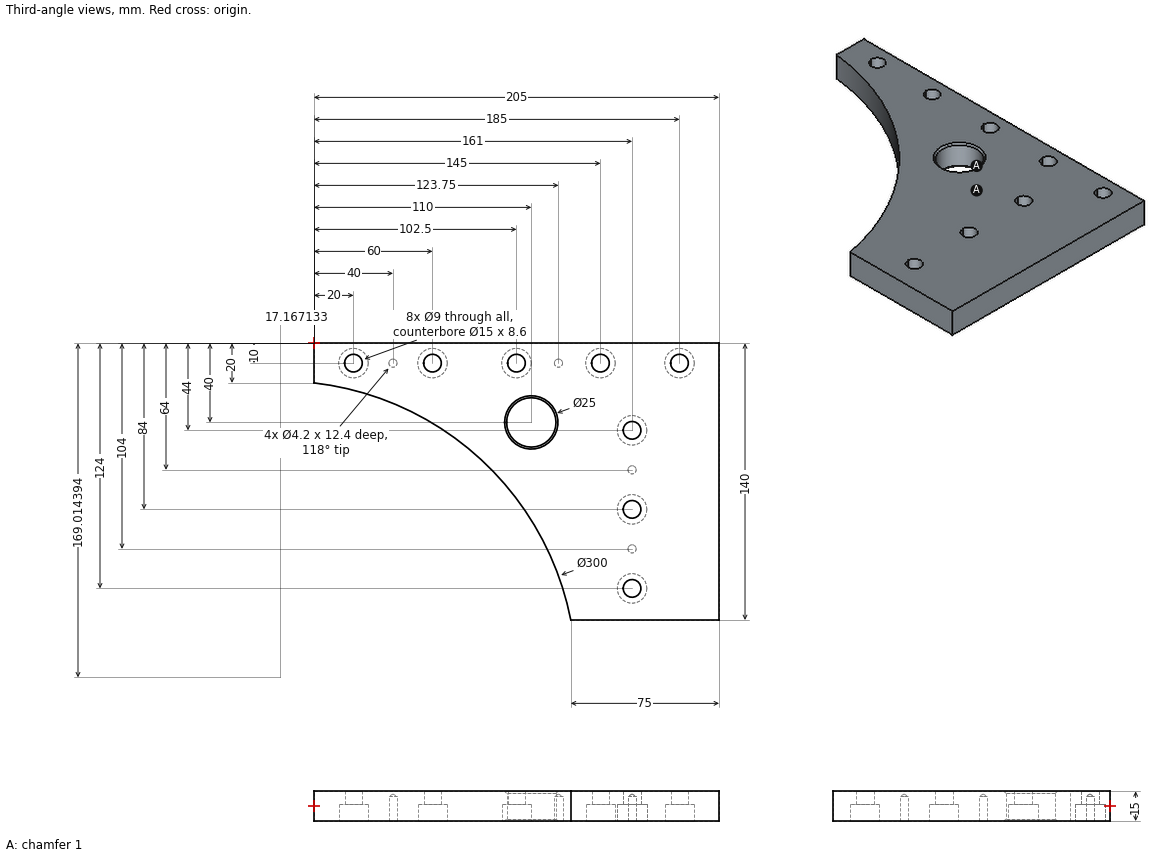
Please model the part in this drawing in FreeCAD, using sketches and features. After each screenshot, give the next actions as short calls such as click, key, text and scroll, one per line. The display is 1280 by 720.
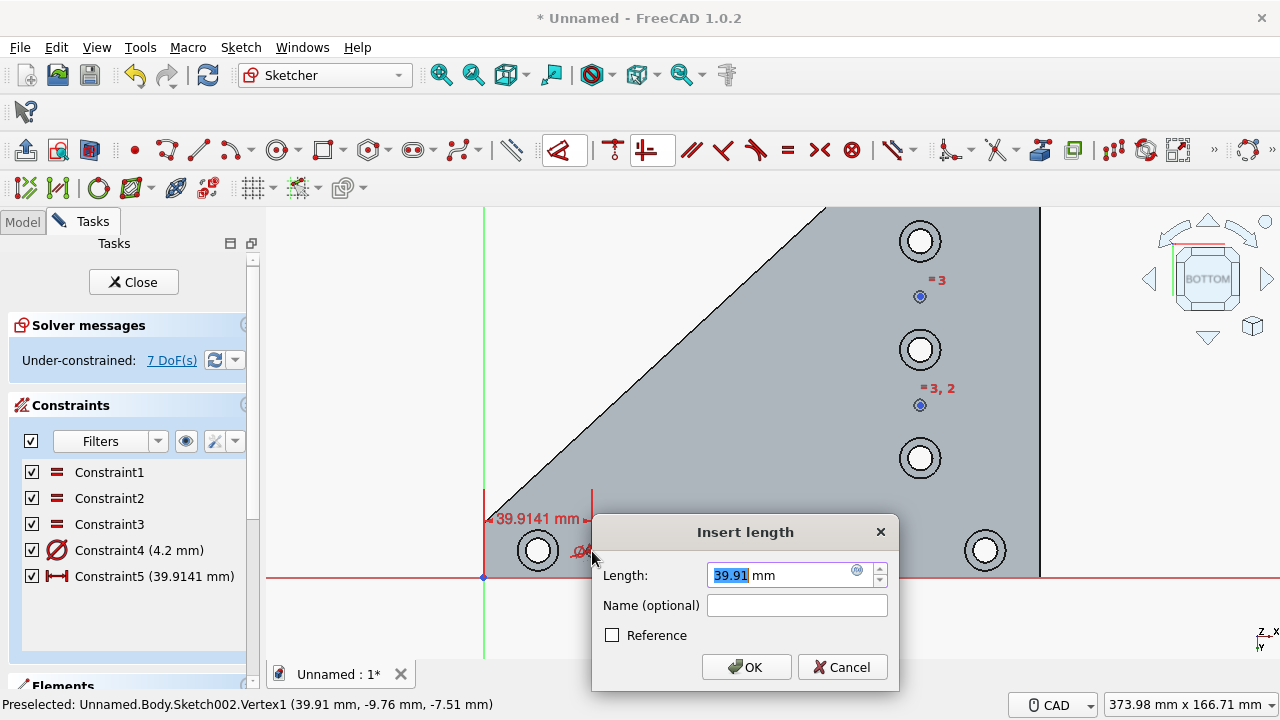
text(40)
key(Return)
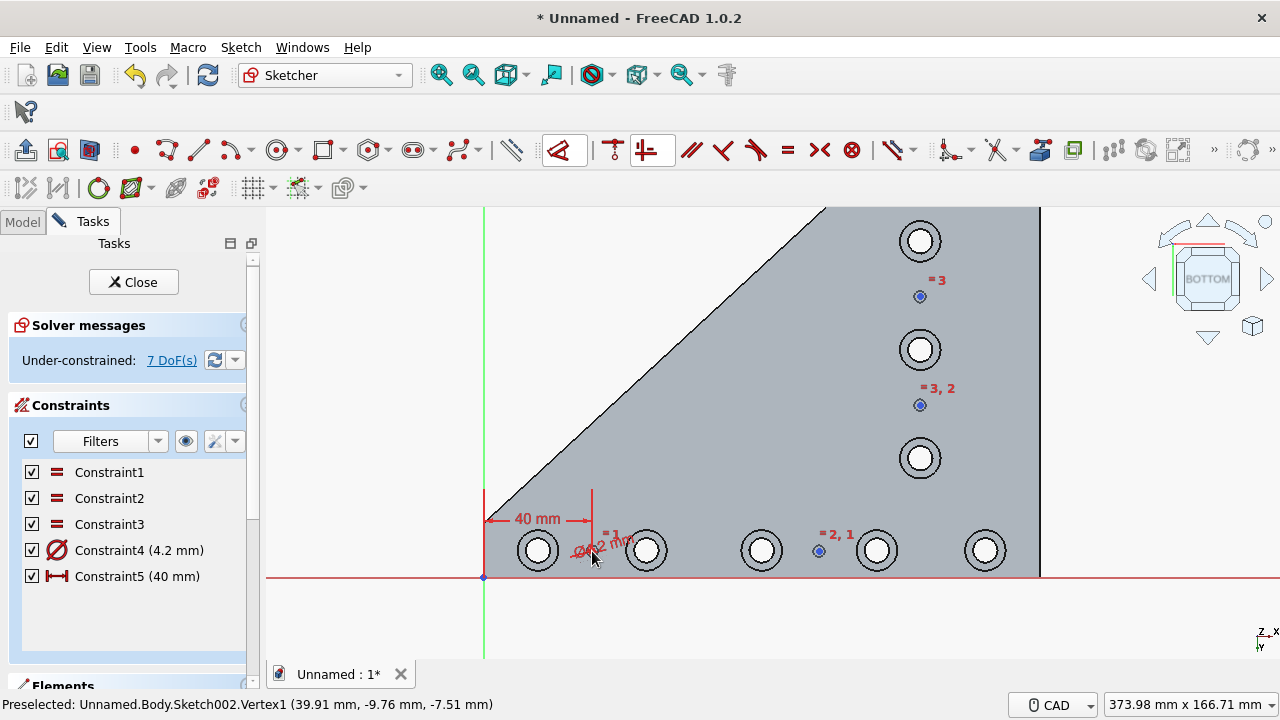
scroll(592, 551, up, 2)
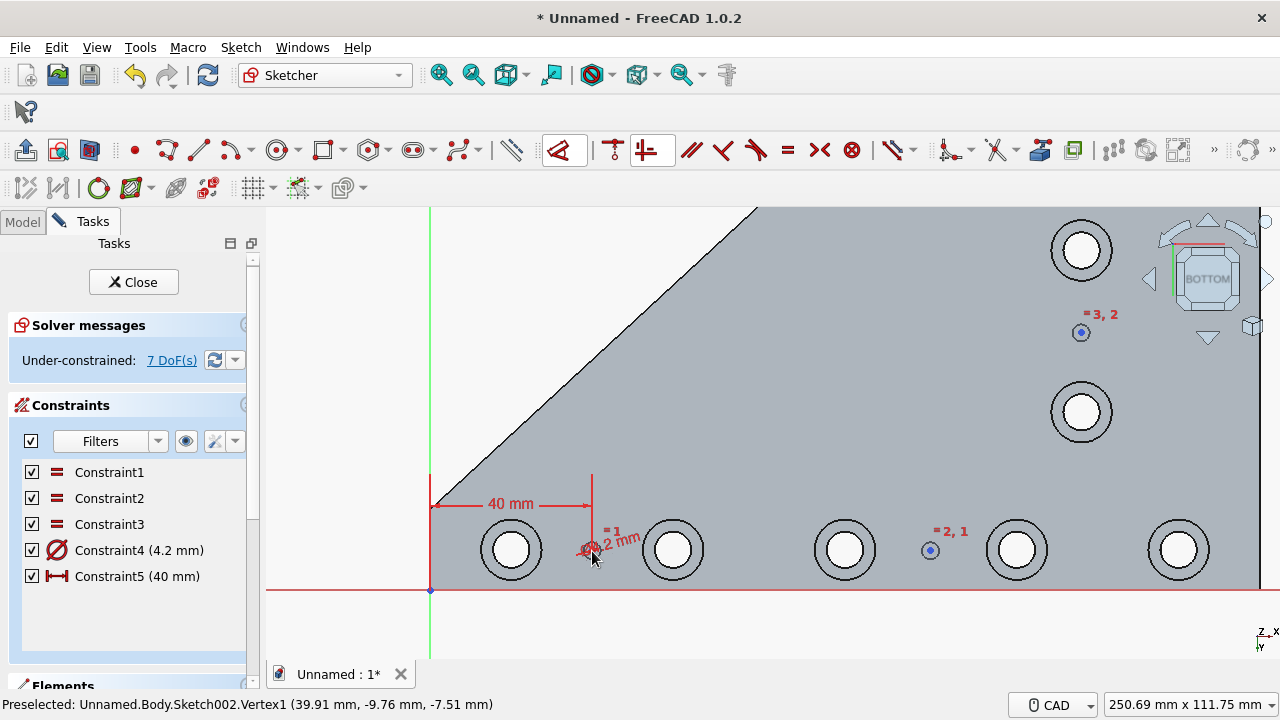
click(592, 551)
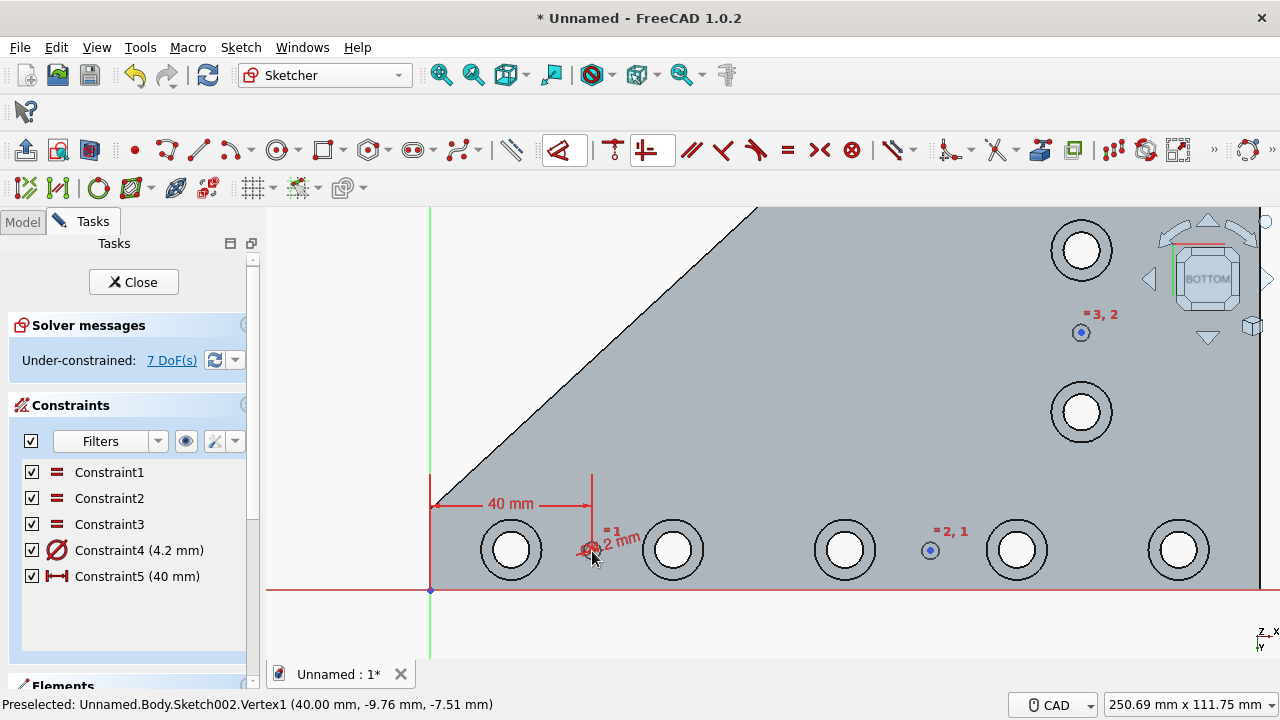
click(582, 150)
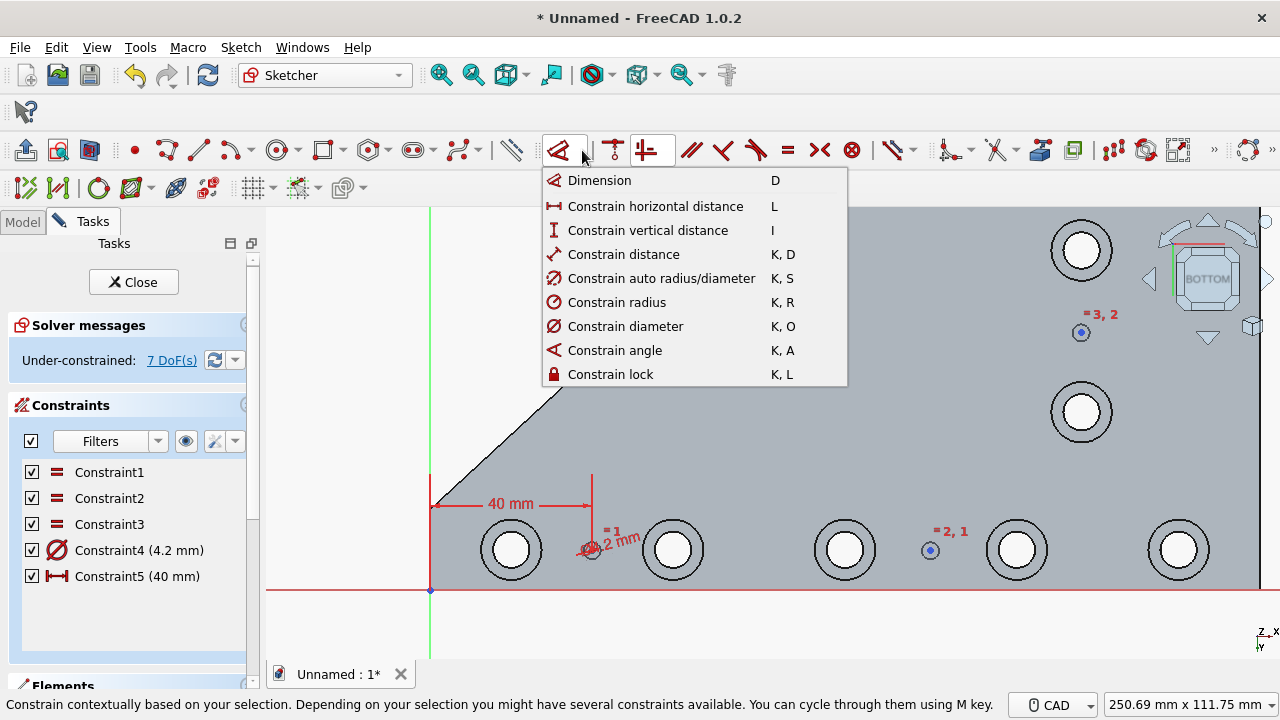
click(695, 230)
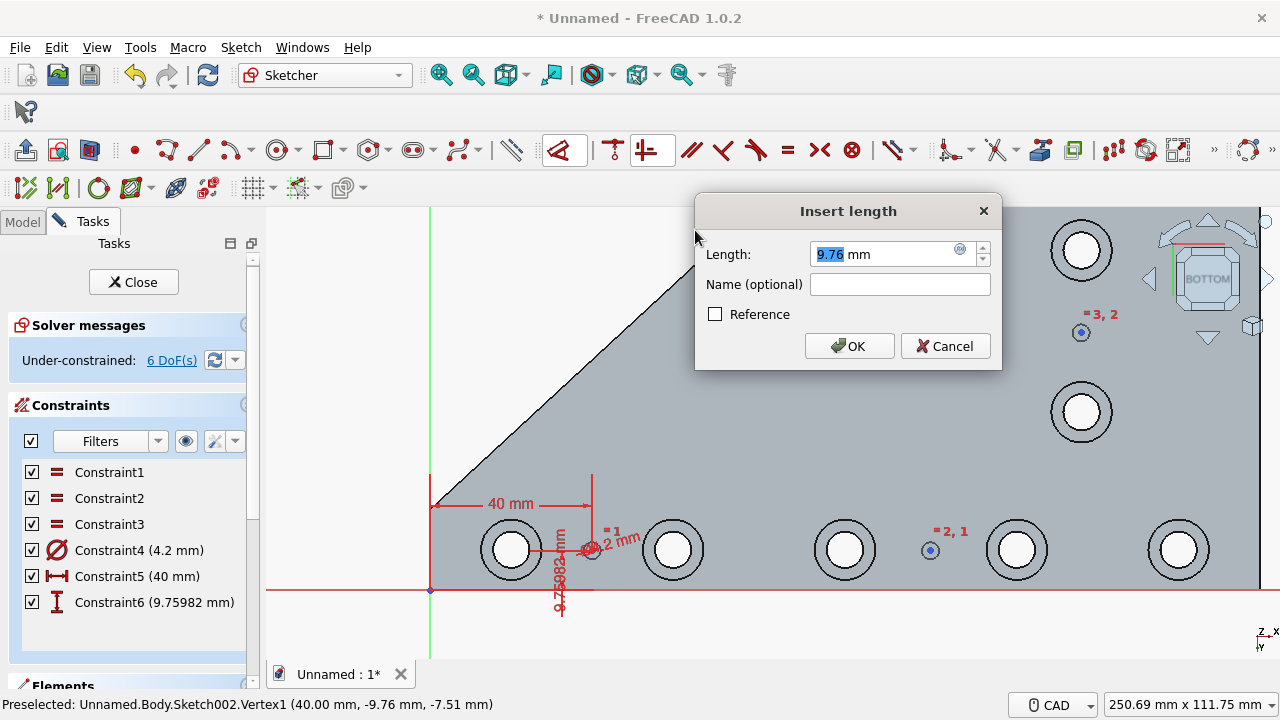
text(10)
key(Return)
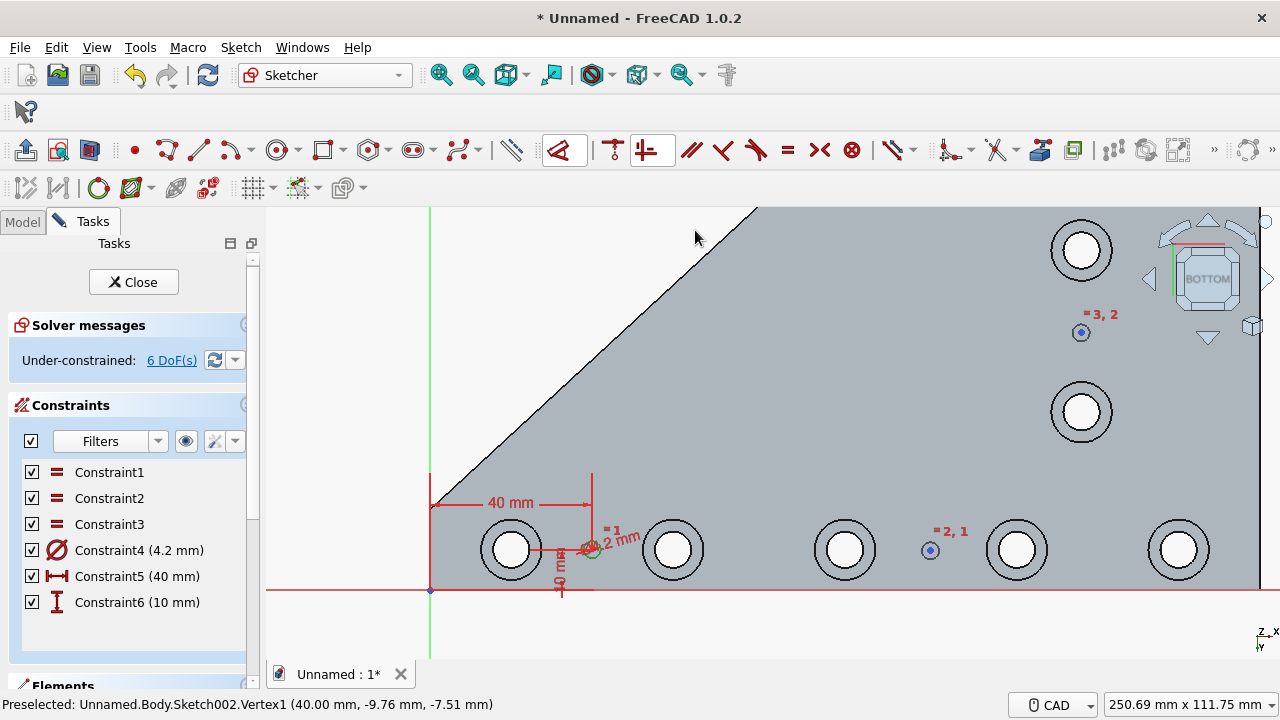
click(930, 551)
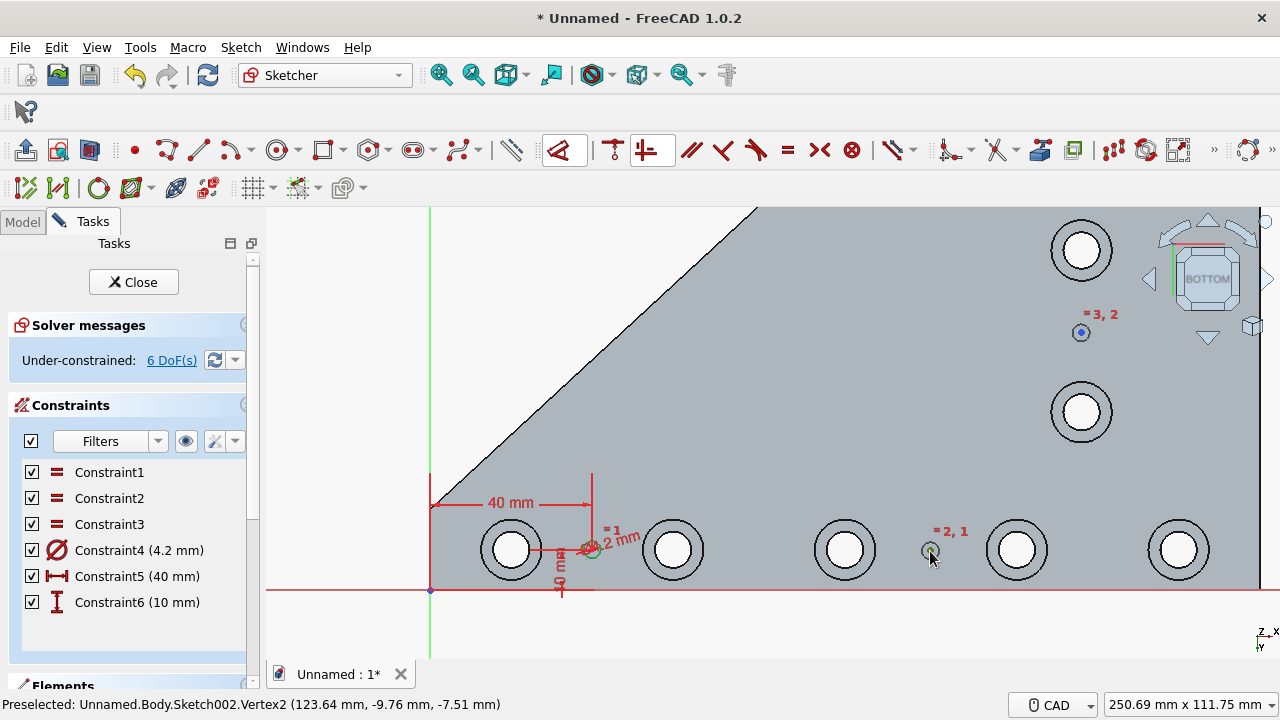
key(i)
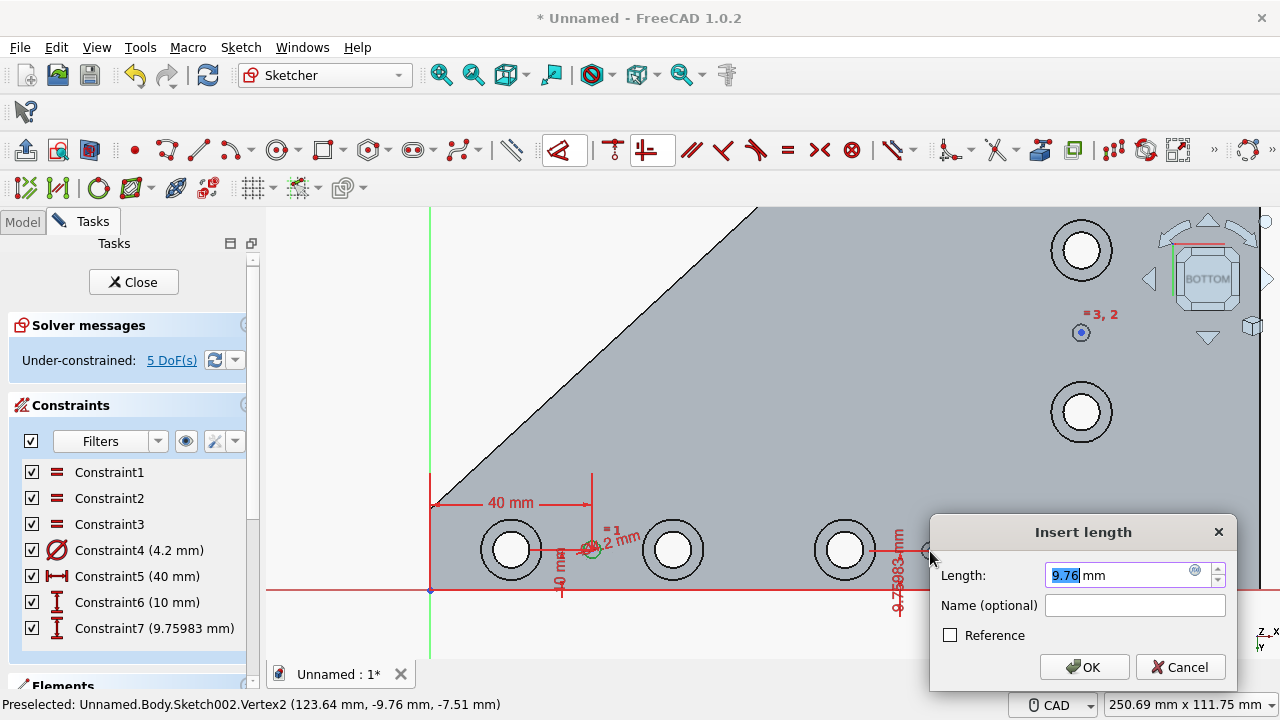
text(10)
key(Return)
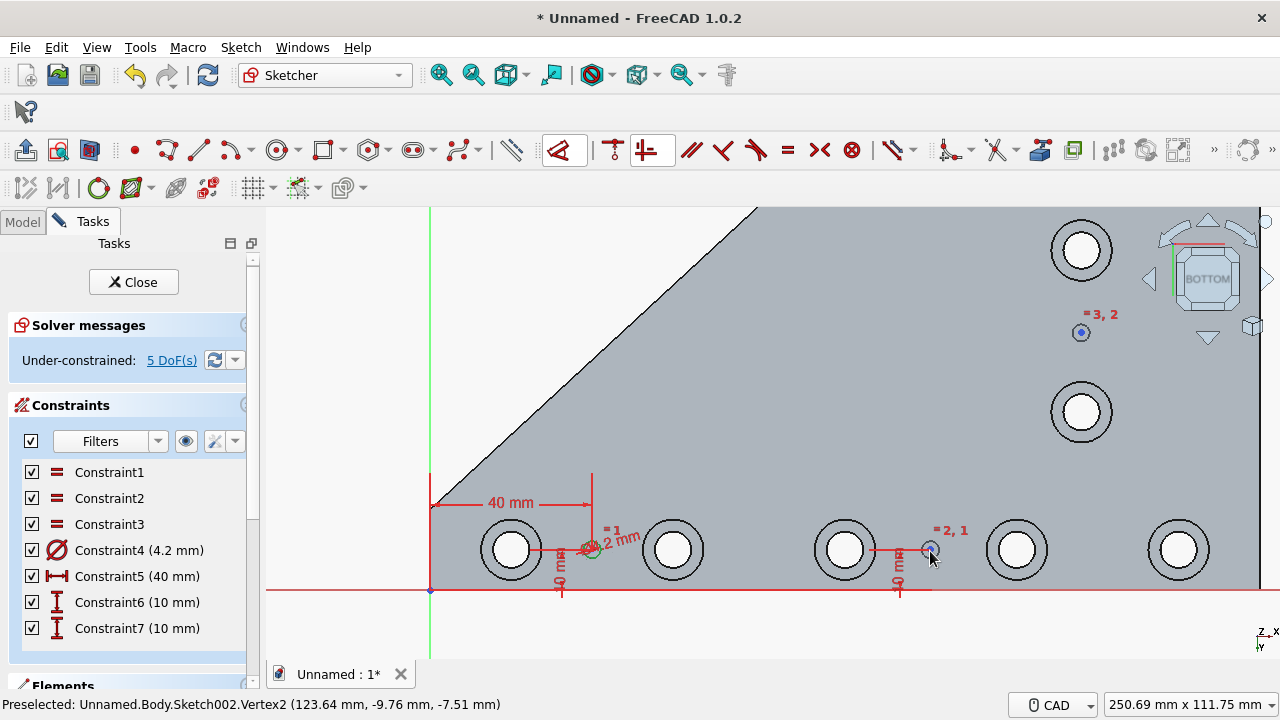
click(1081, 333)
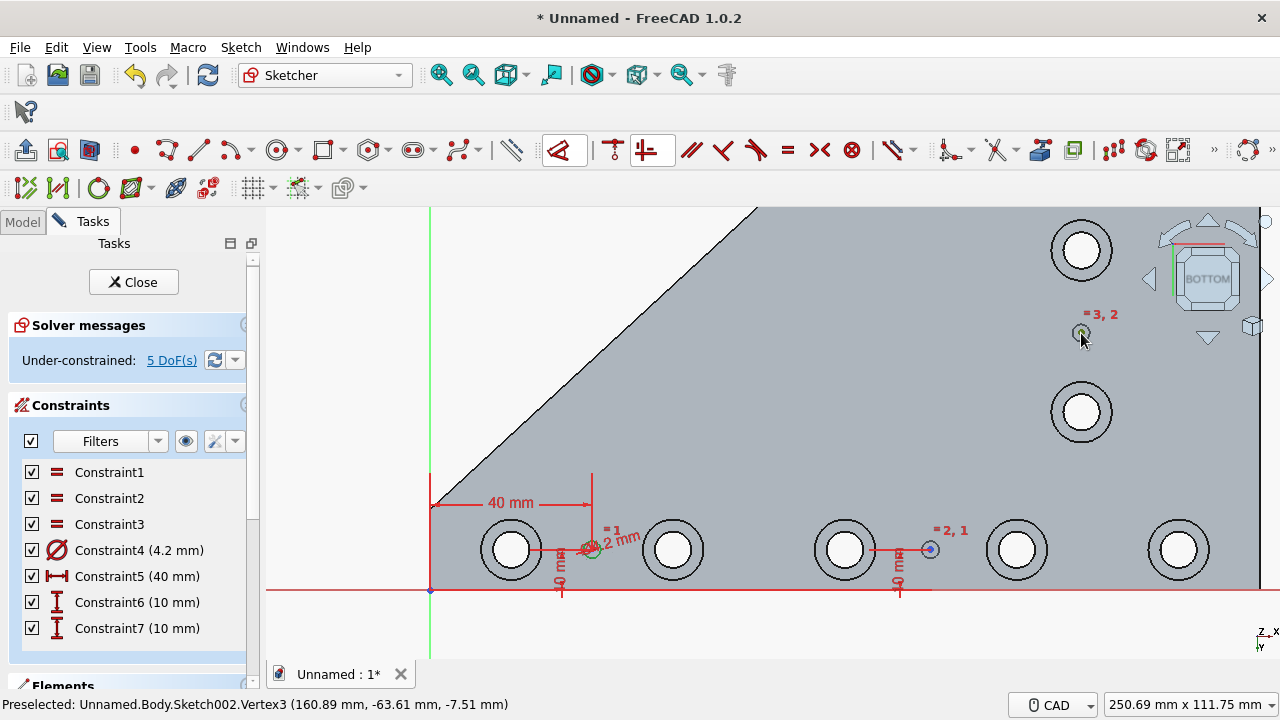
click(582, 150)